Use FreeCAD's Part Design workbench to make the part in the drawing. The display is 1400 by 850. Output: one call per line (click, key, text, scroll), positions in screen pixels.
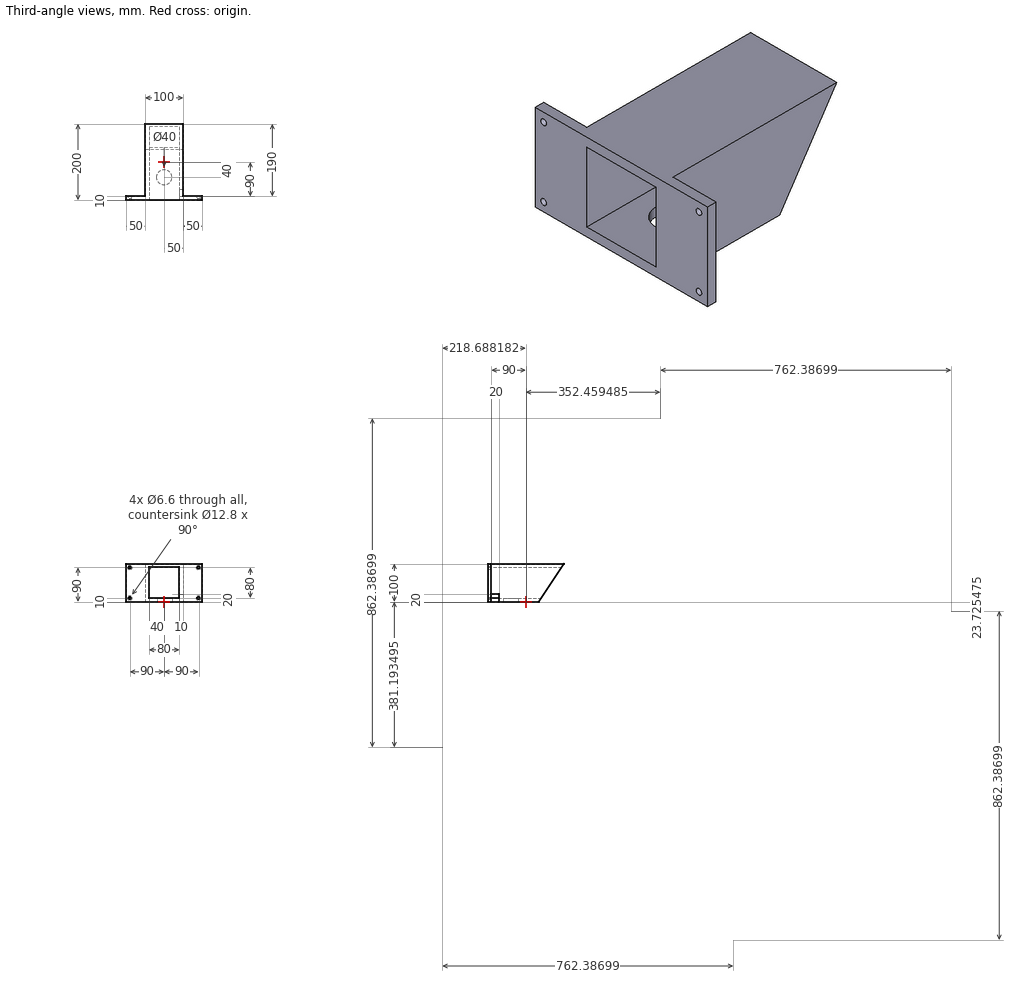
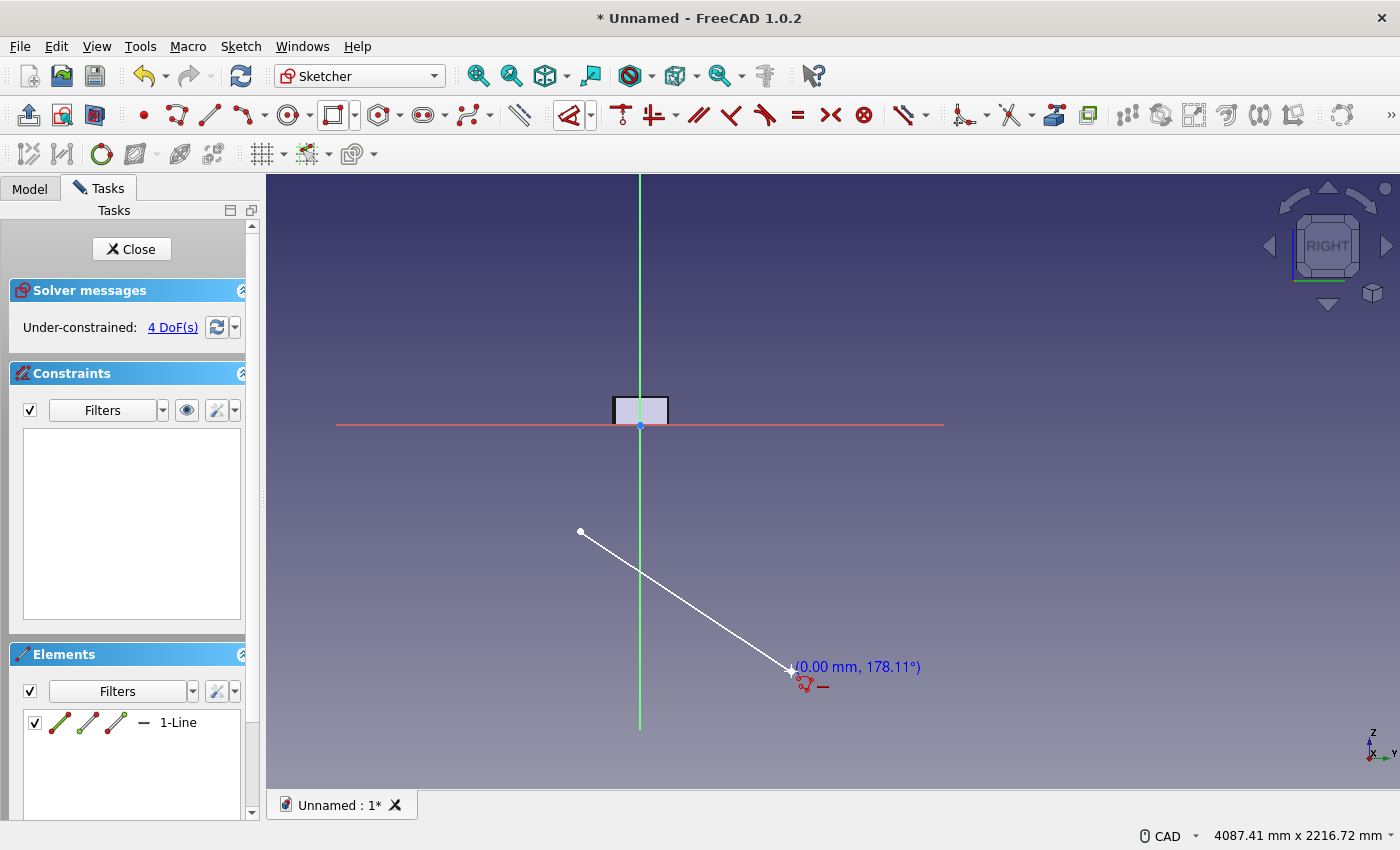
scroll(950, 432, up, 5)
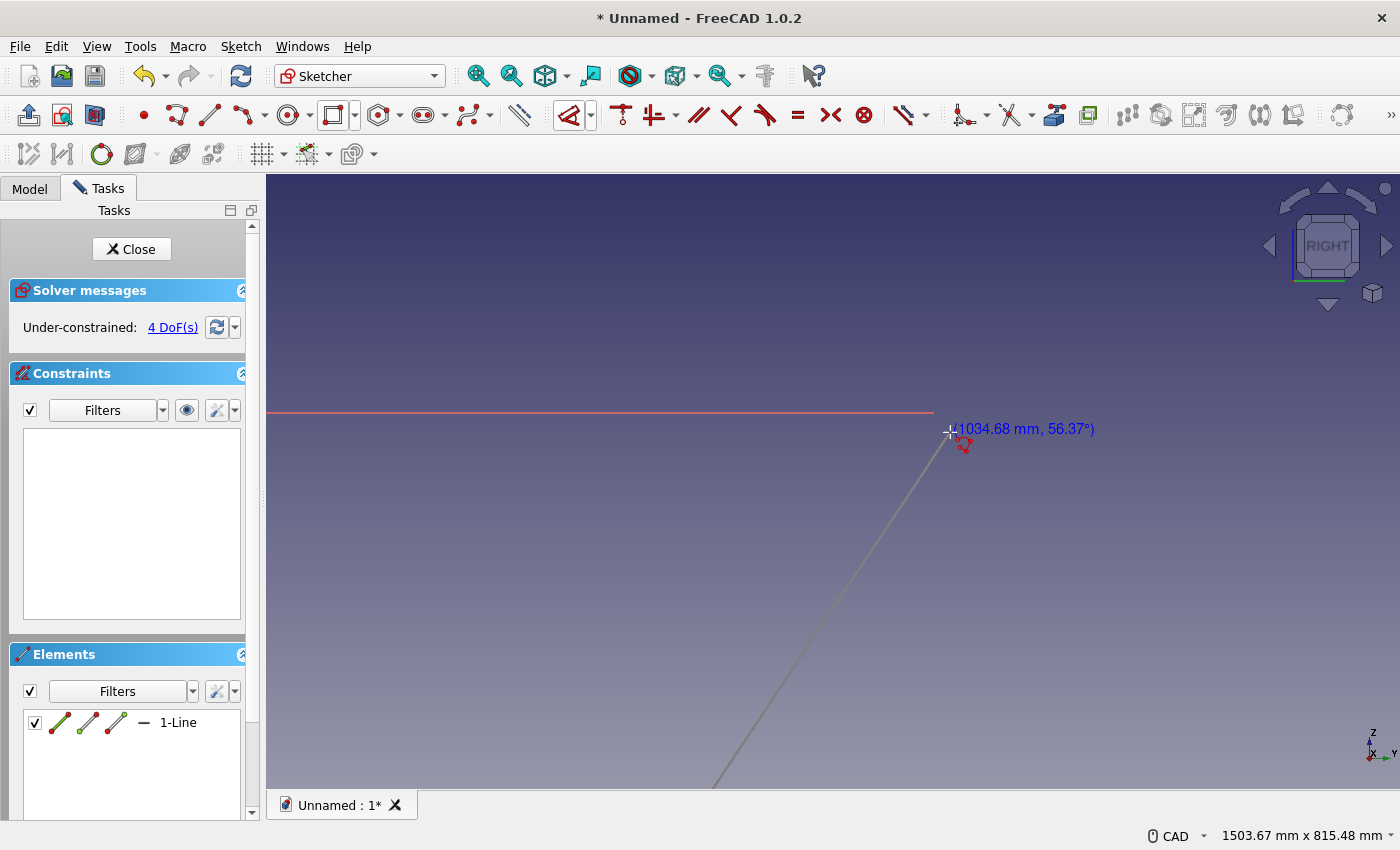
click(948, 431)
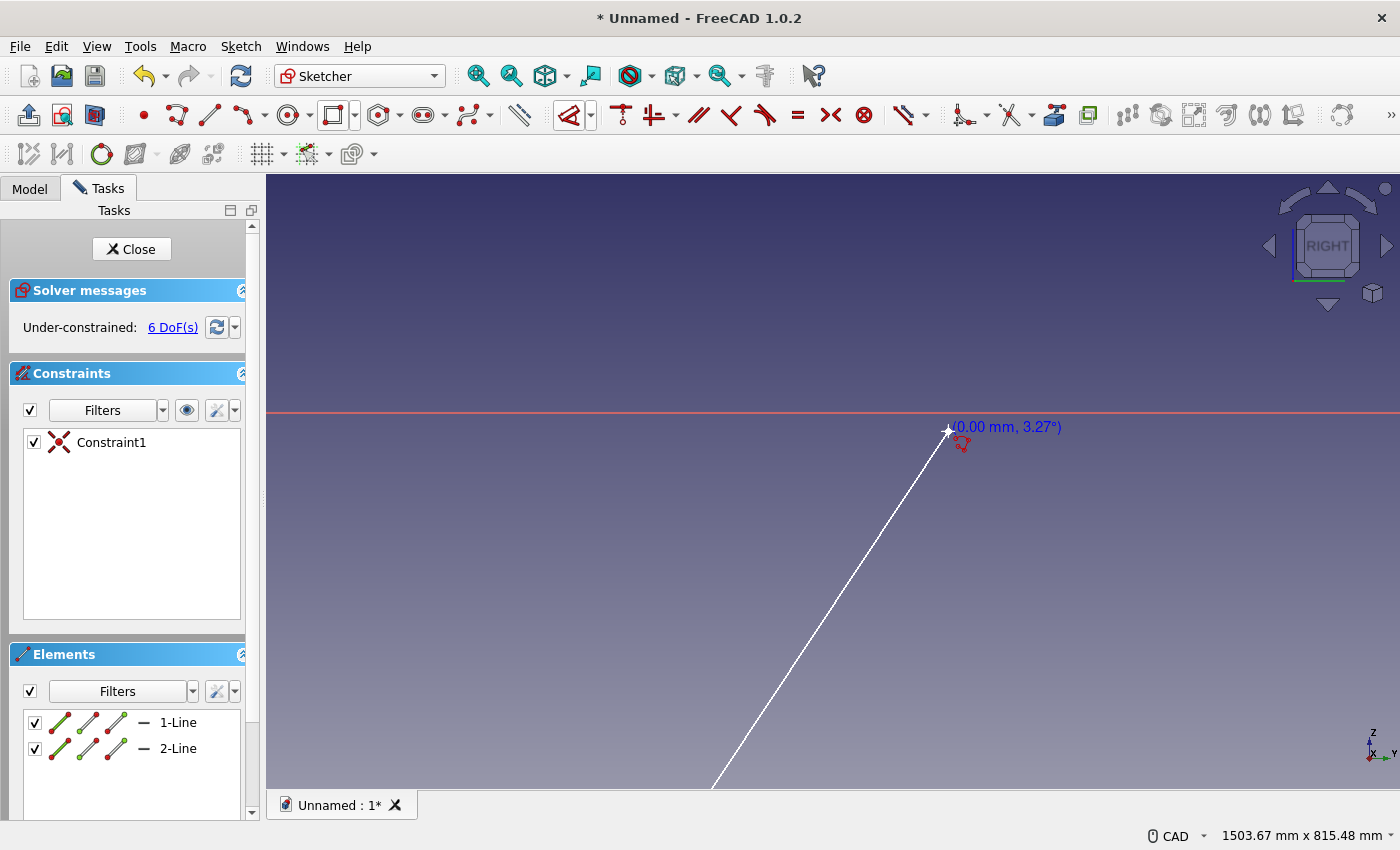
scroll(950, 433, down, 5)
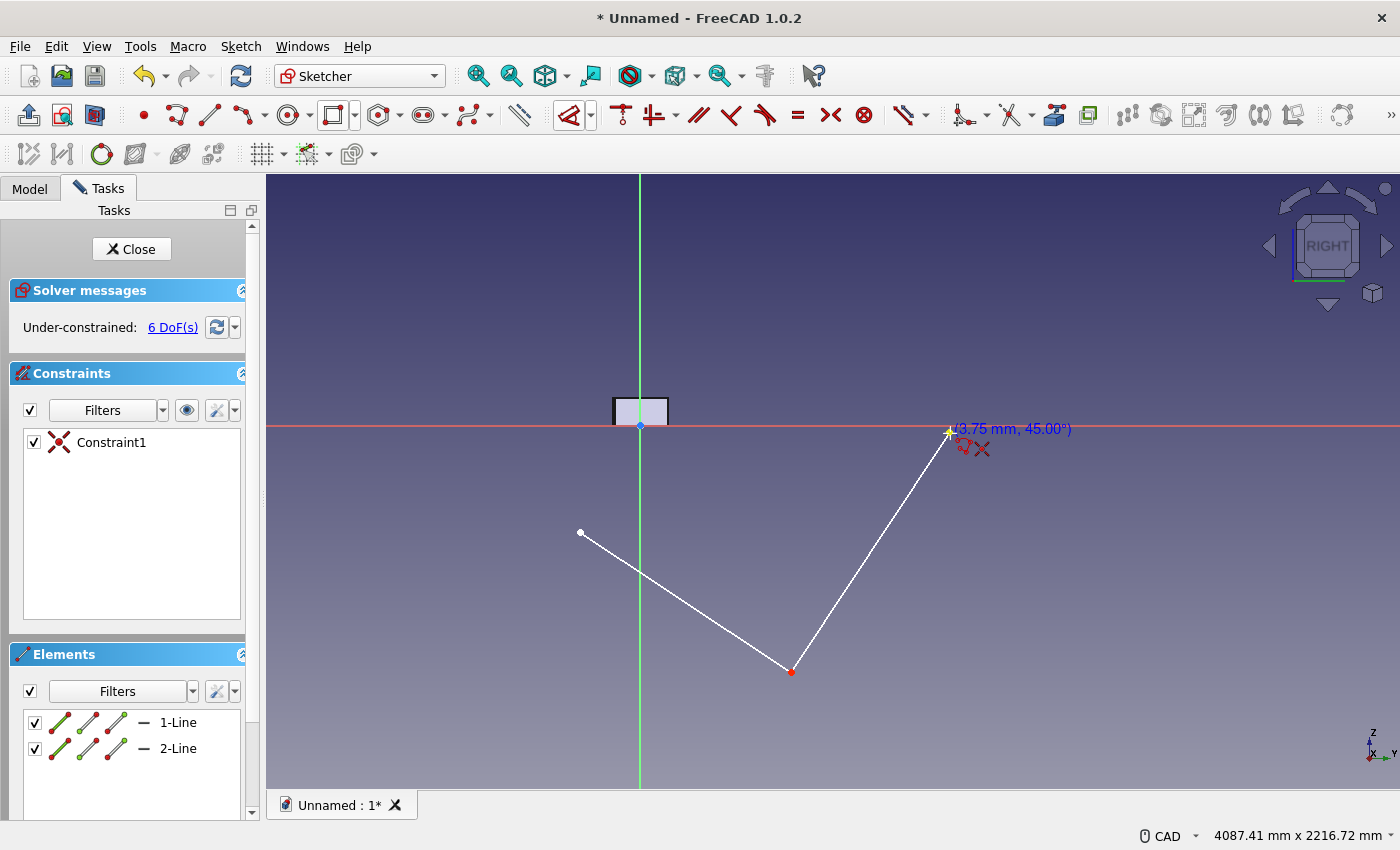
click(738, 292)
click(580, 533)
key(Escape)
key(Escape)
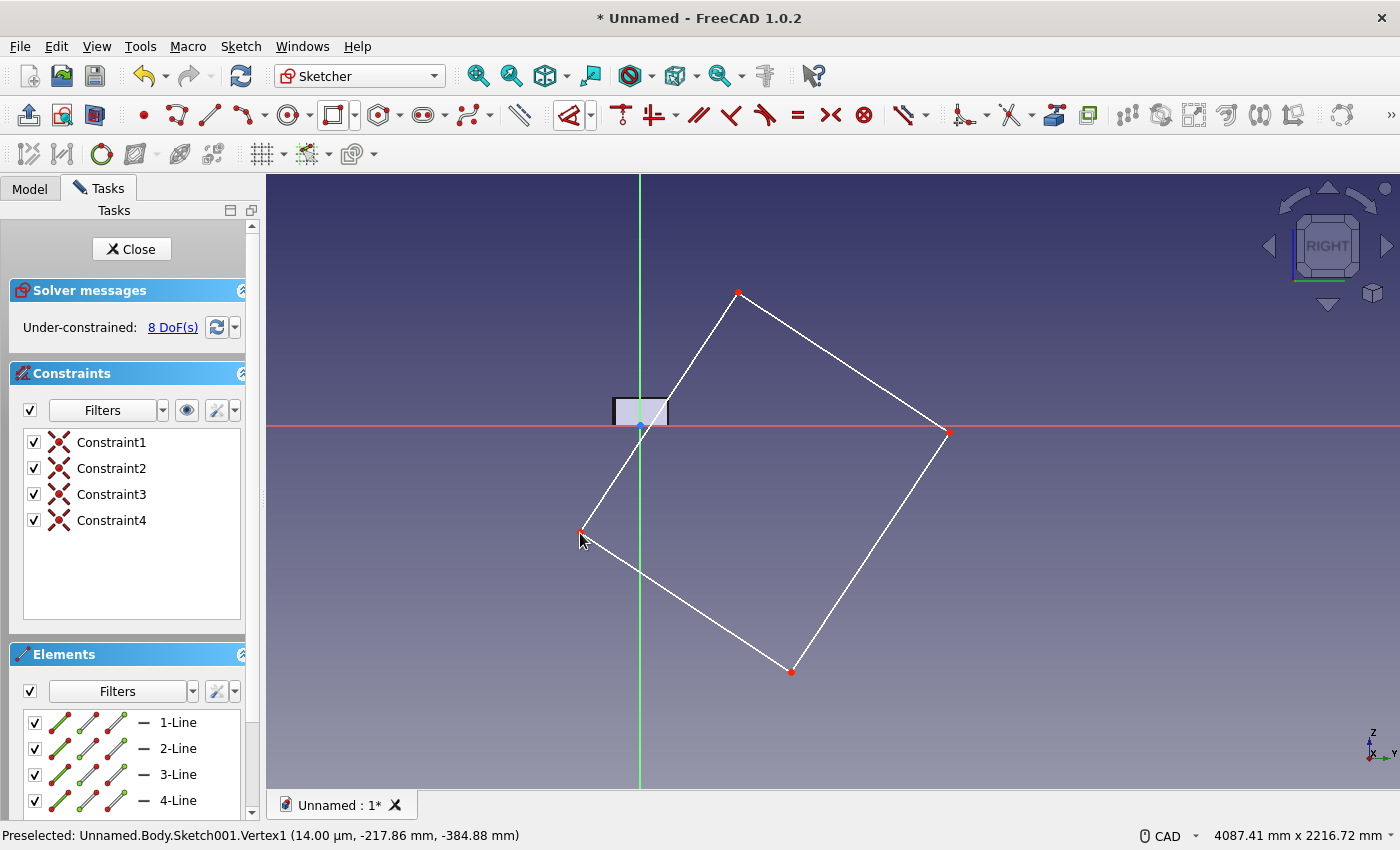
click(568, 116)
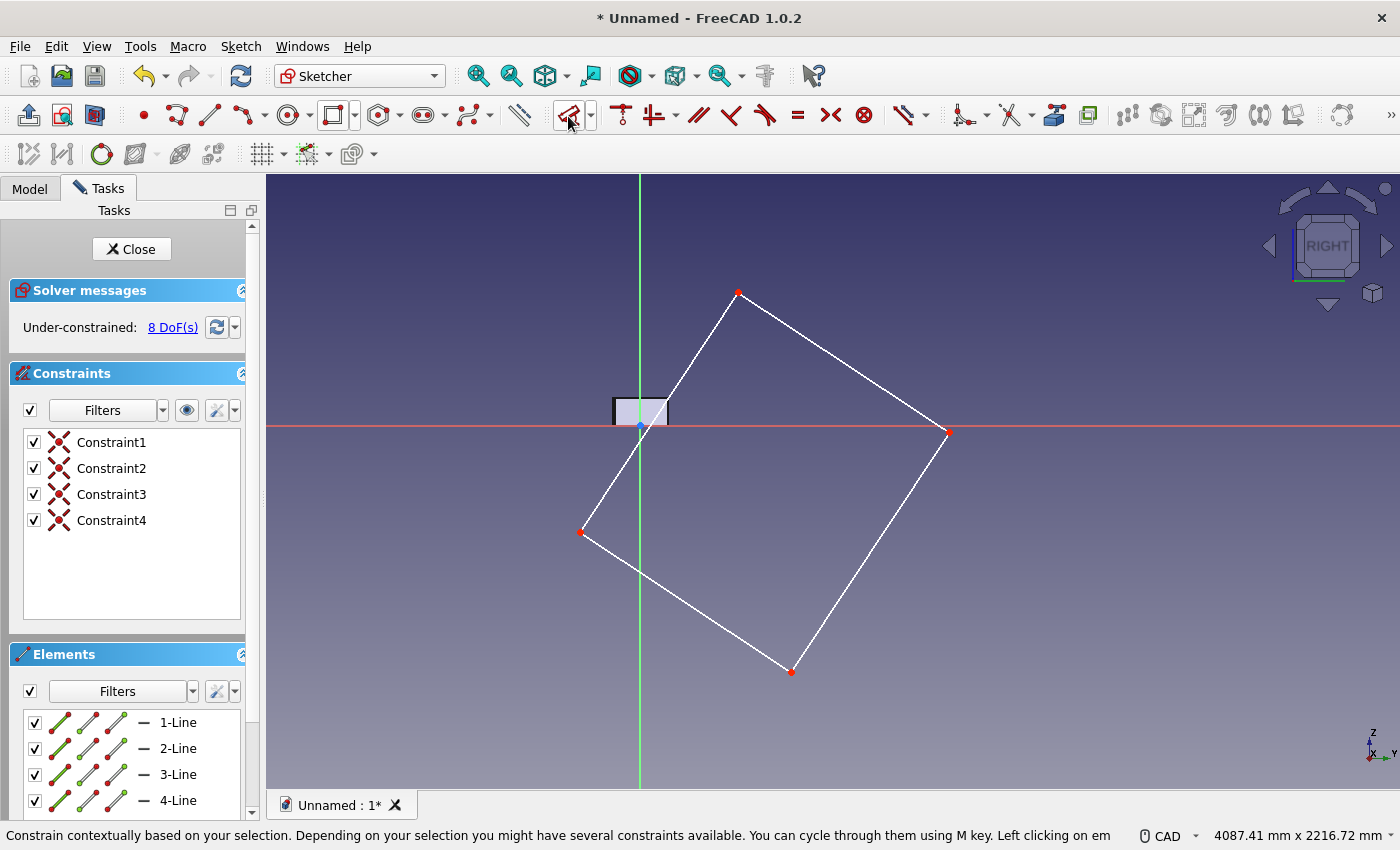
scroll(950, 433, up, 9)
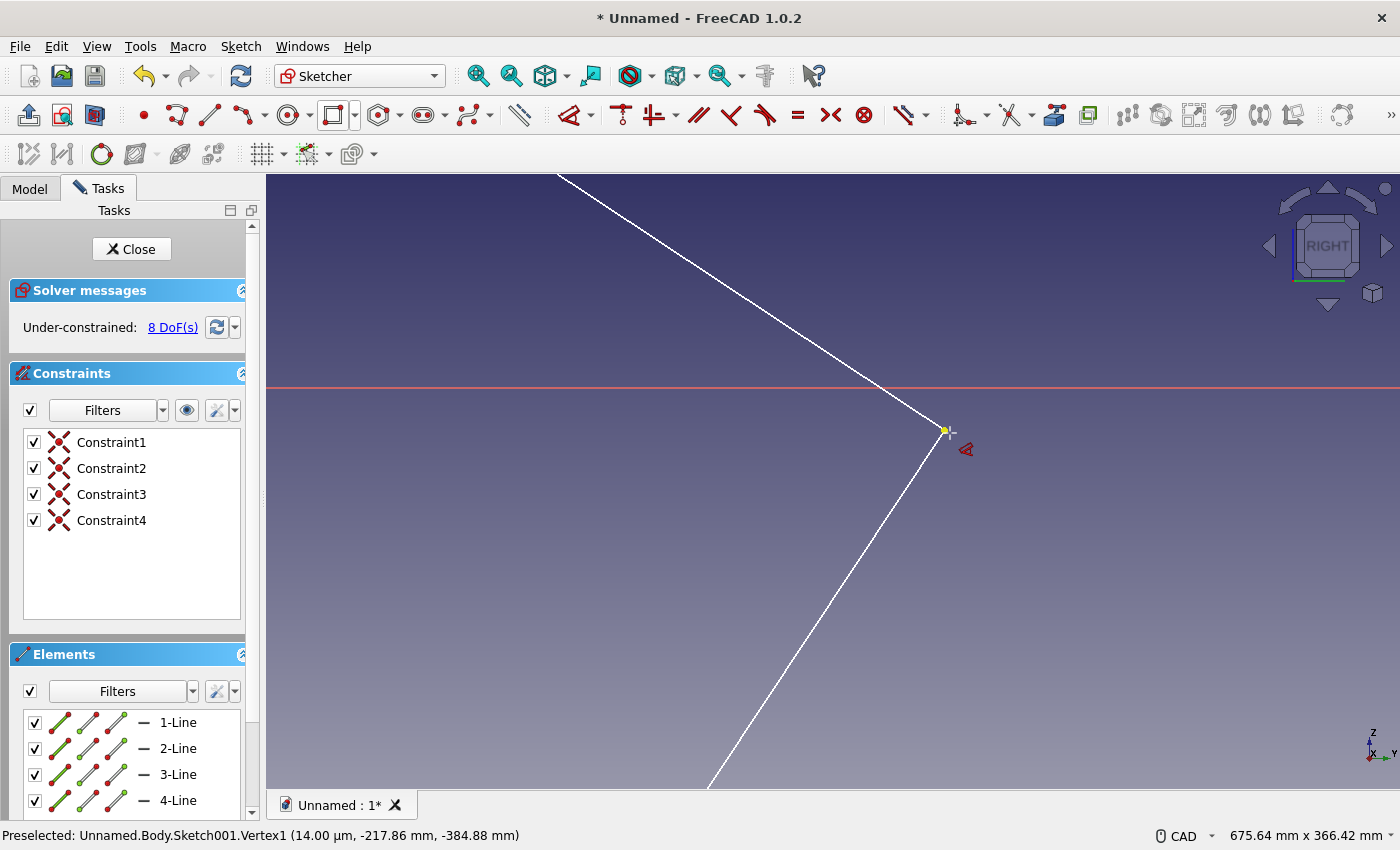
click(945, 430)
click(979, 409)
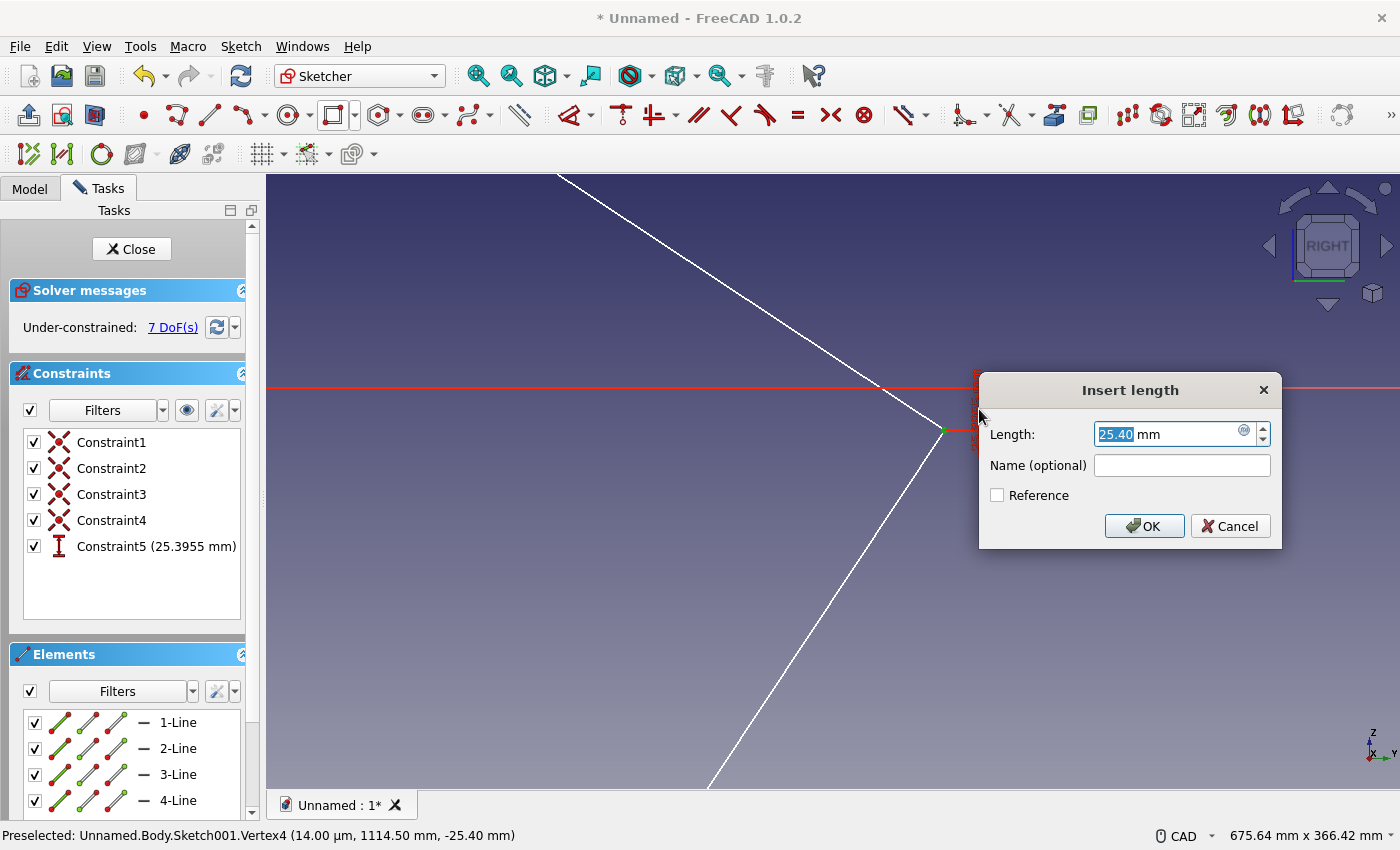
text(23.725475)
key(Return)